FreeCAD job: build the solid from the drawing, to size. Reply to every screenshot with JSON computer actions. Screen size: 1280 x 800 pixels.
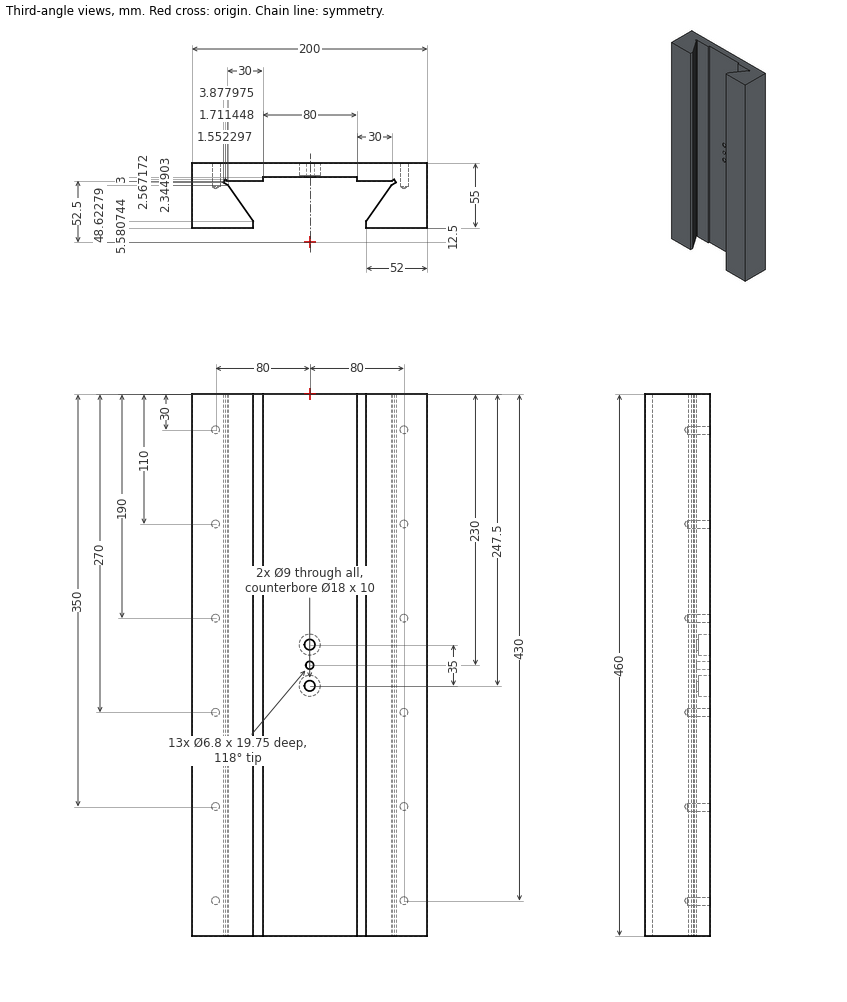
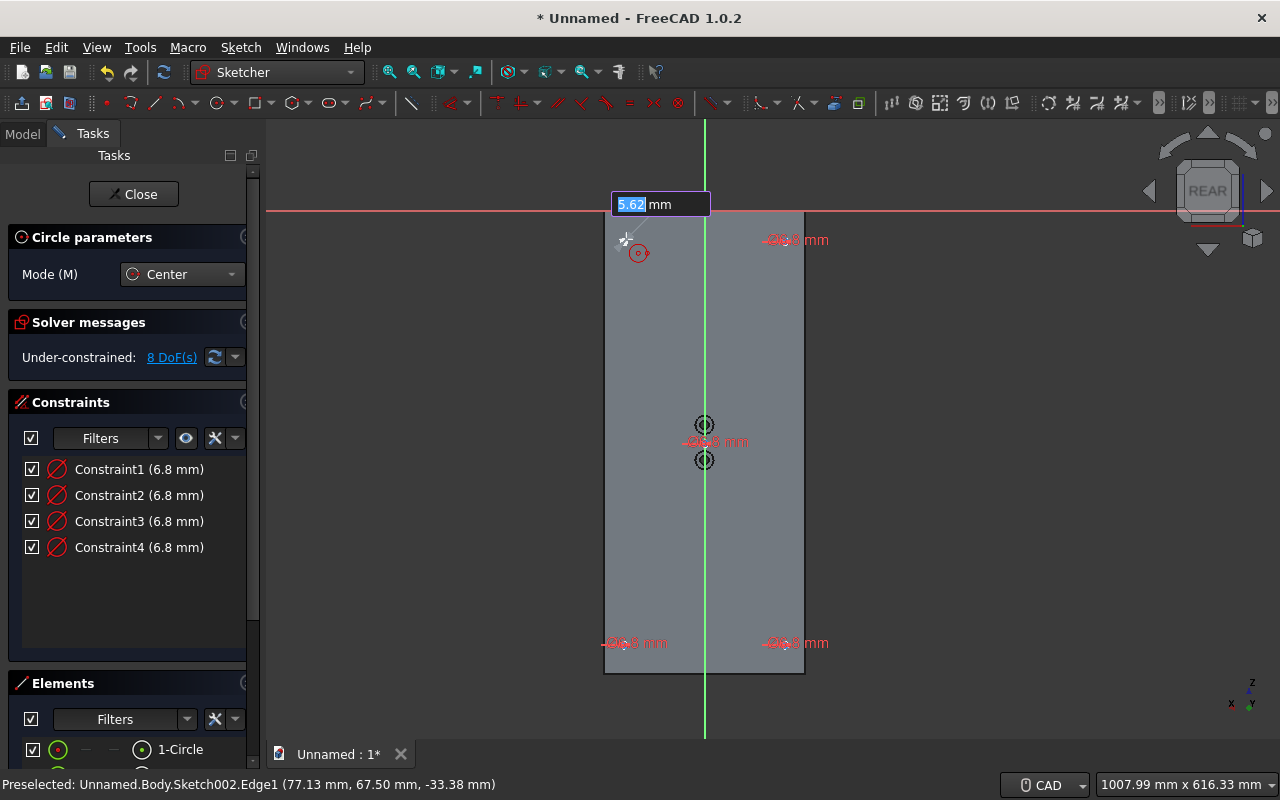
{"action": "type", "text": "6.8"}
{"action": "key", "text": "Return"}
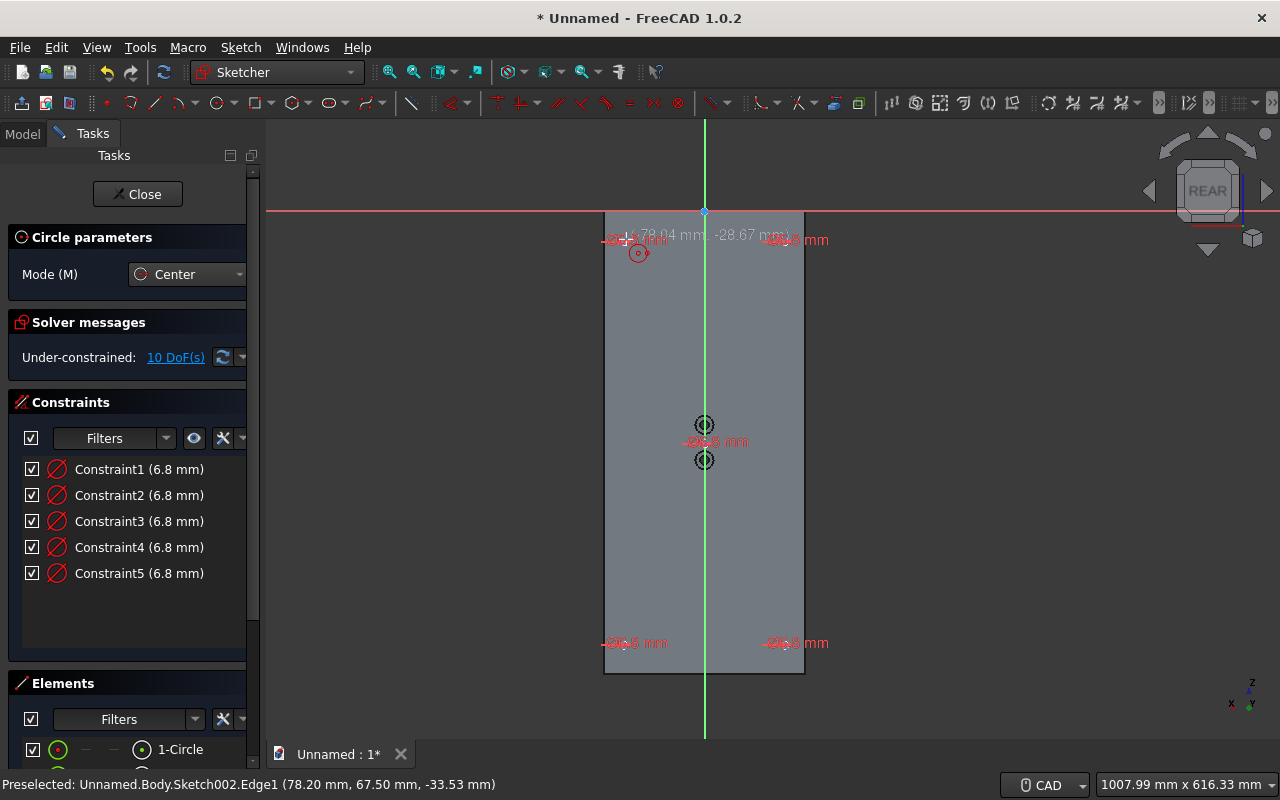
{"action": "scroll", "coordinate": [785, 563], "scroll_direction": "up", "scroll_amount": 10}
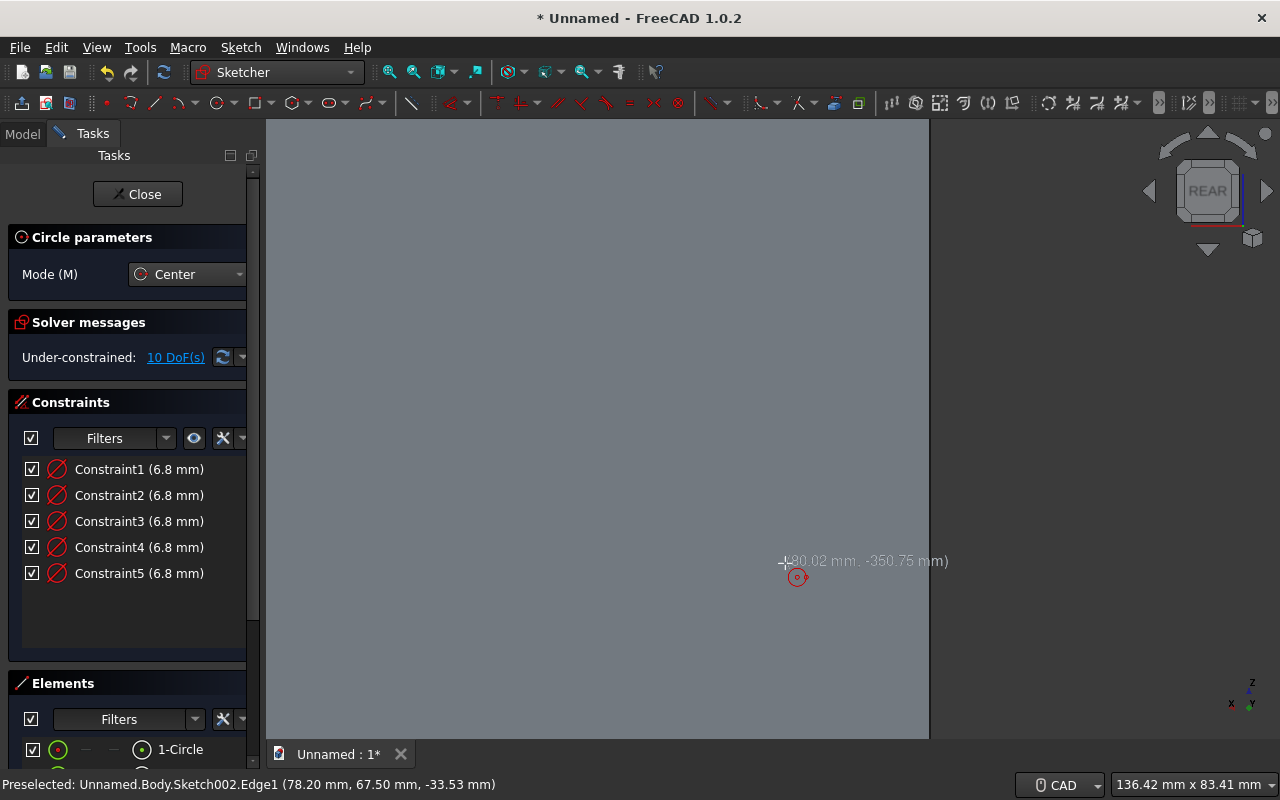
{"action": "scroll", "coordinate": [786, 564], "scroll_direction": "down", "scroll_amount": 10}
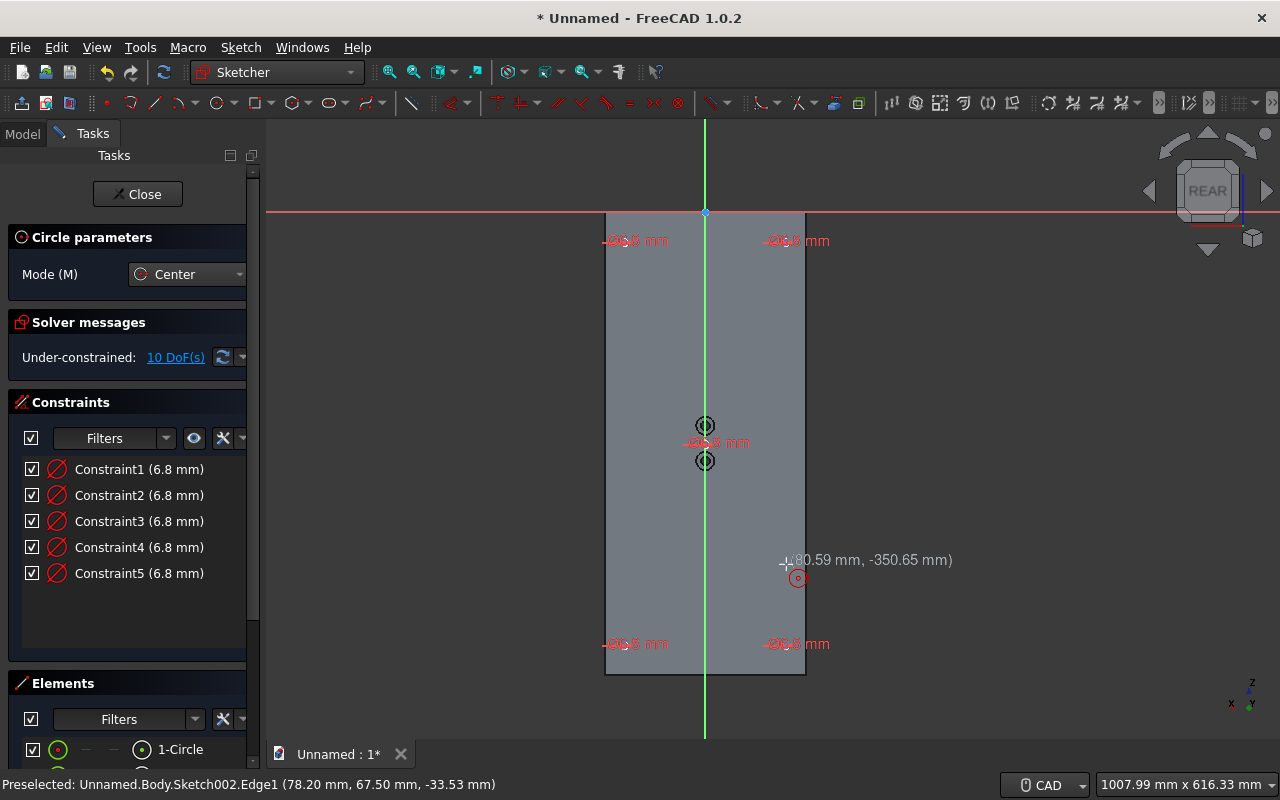
{"action": "left_click", "coordinate": [786, 564]}
{"action": "mouse_move", "coordinate": [788, 562]}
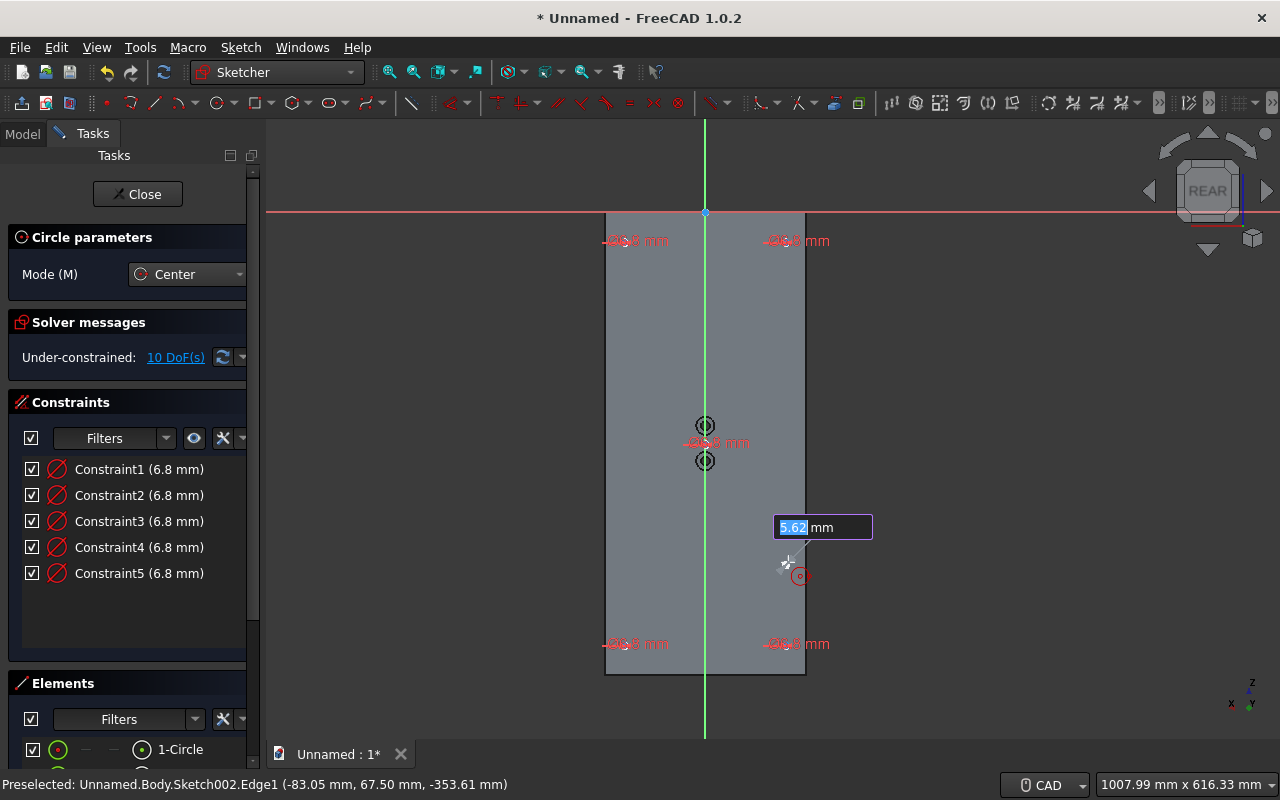
{"action": "type", "text": "6.8"}
{"action": "key", "text": "Return"}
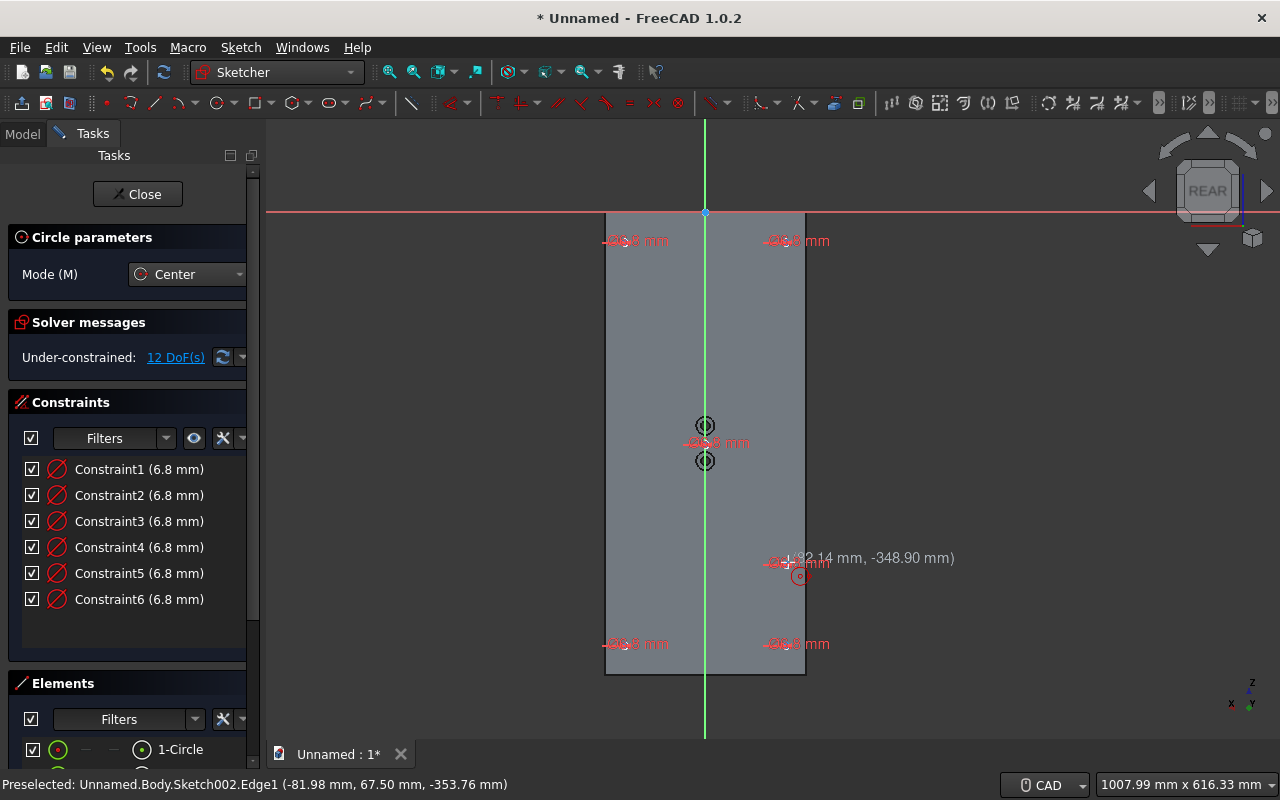
{"action": "scroll", "coordinate": [625, 564], "scroll_direction": "up", "scroll_amount": 10}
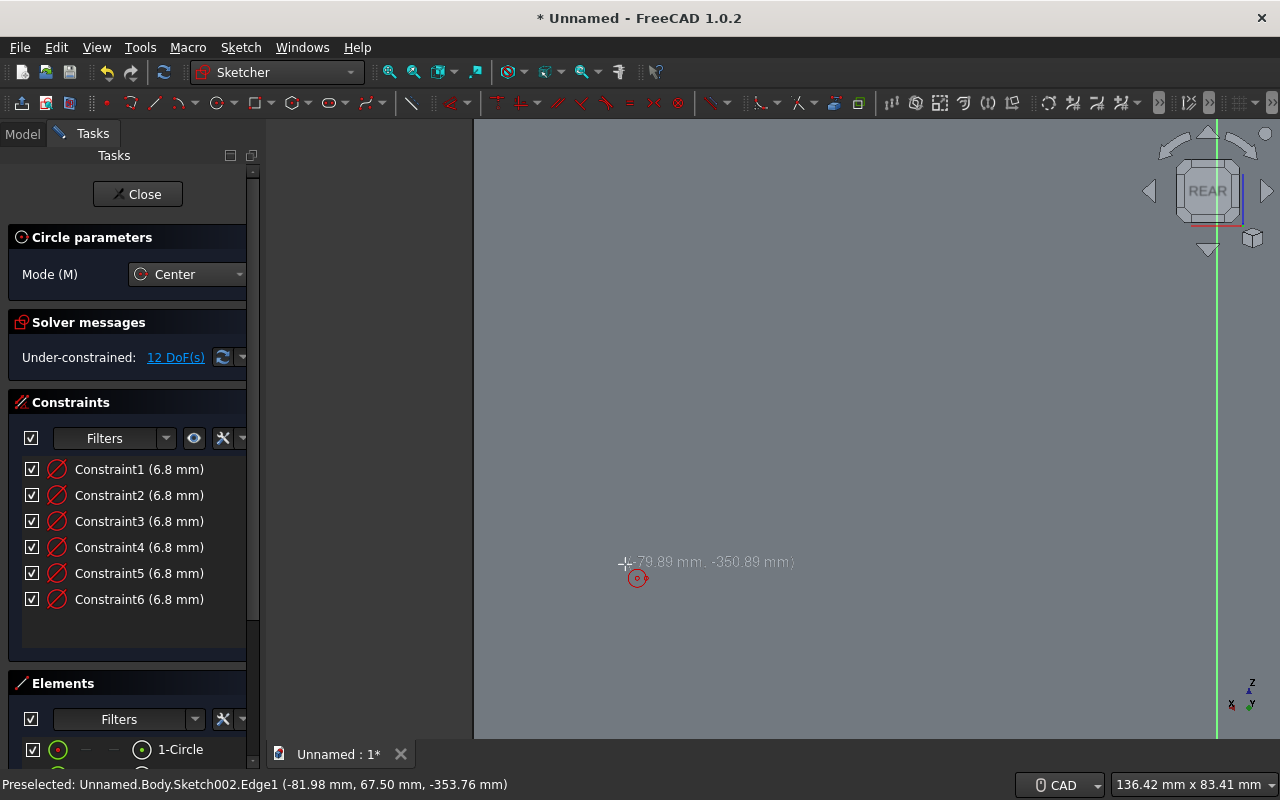
{"action": "scroll", "coordinate": [624, 564], "scroll_direction": "down", "scroll_amount": 10}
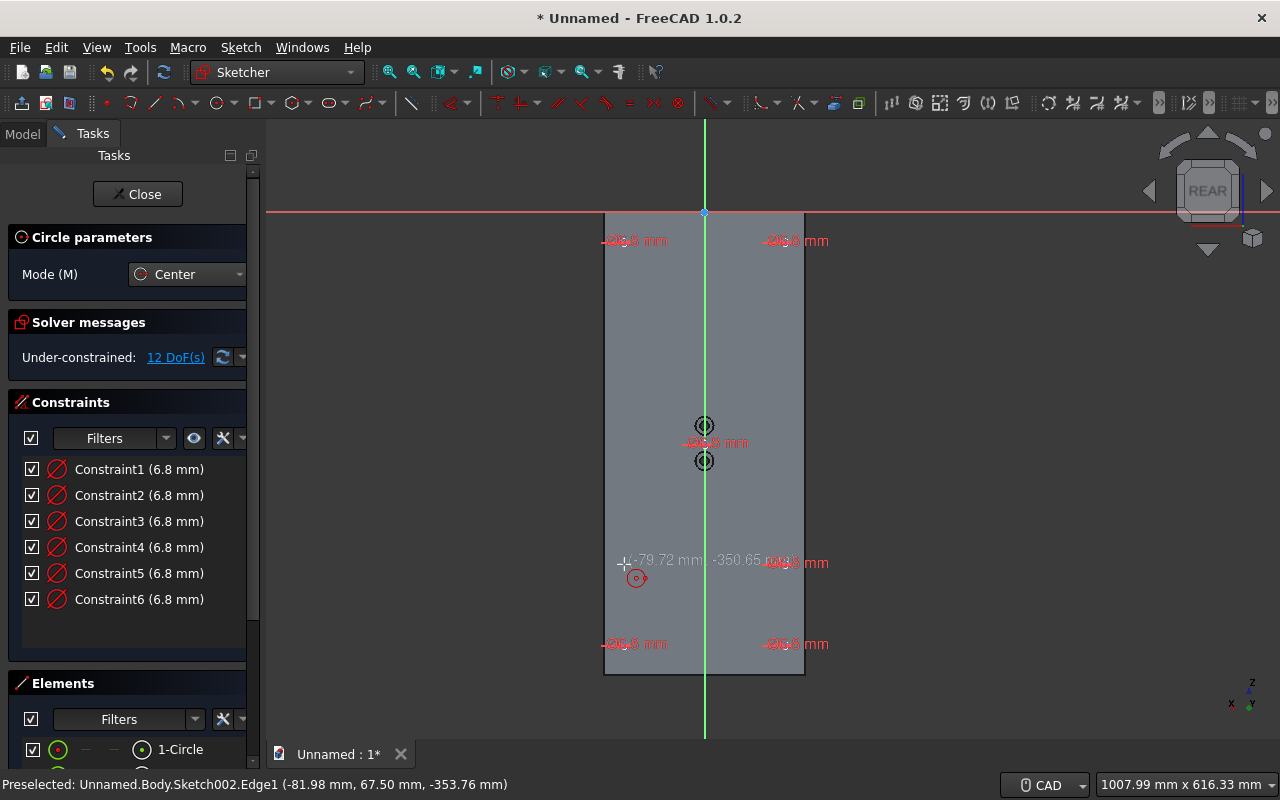
{"action": "left_click", "coordinate": [624, 564]}
{"action": "mouse_move", "coordinate": [626, 562]}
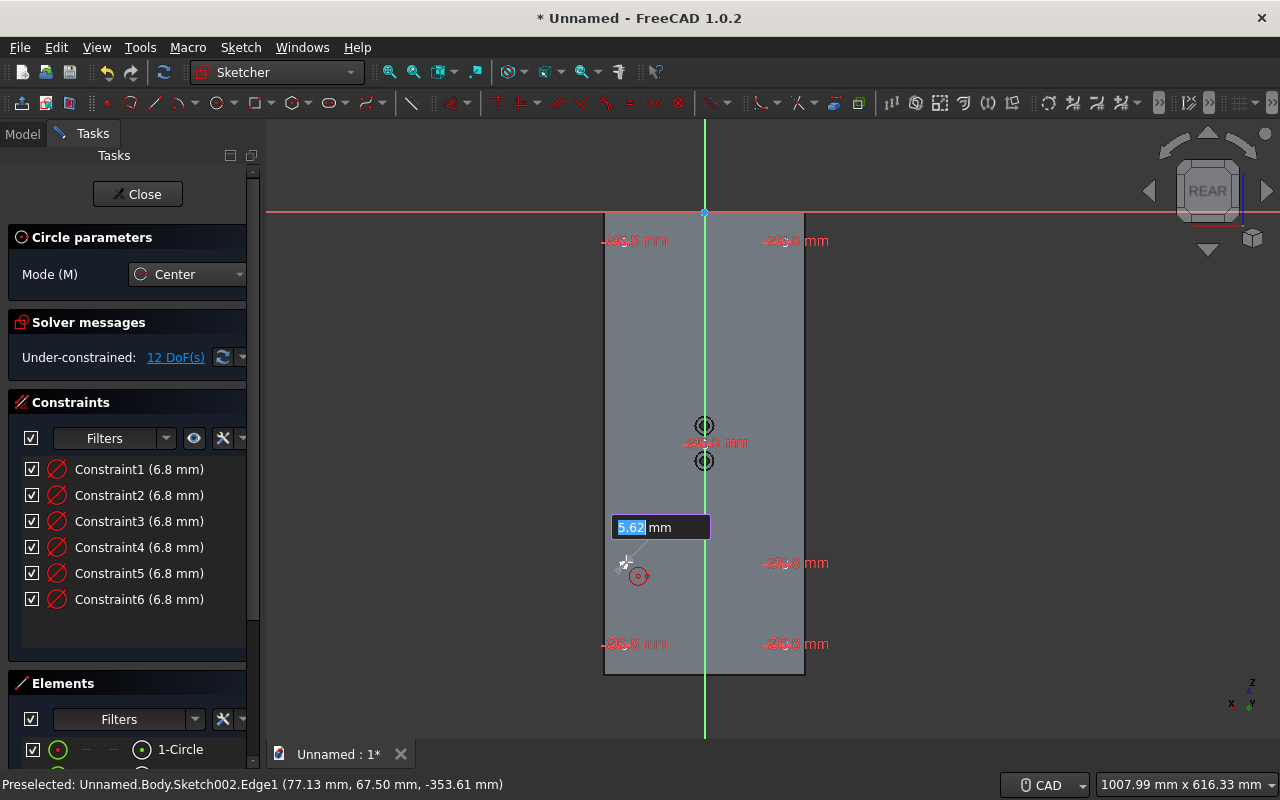
{"action": "type", "text": "6.8"}
{"action": "key", "text": "Return"}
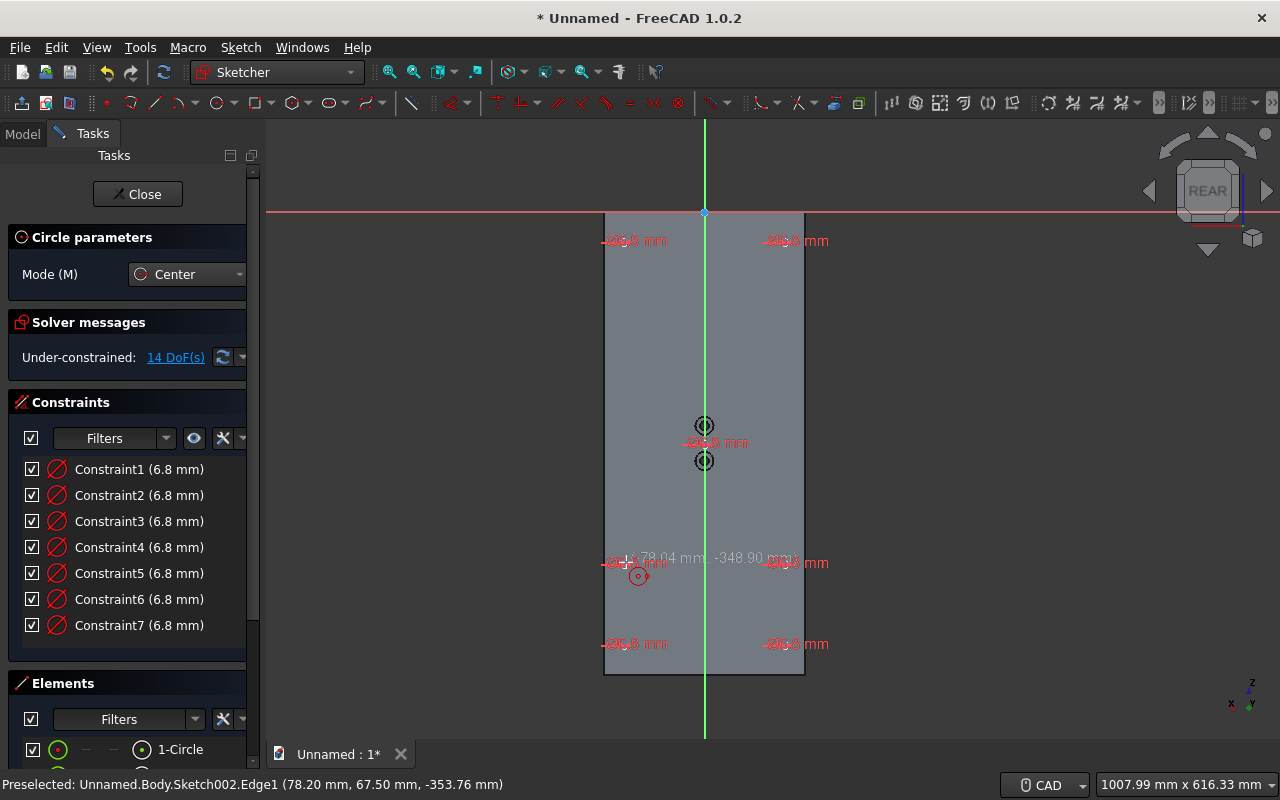
{"action": "scroll", "coordinate": [785, 484], "scroll_direction": "up", "scroll_amount": 10}